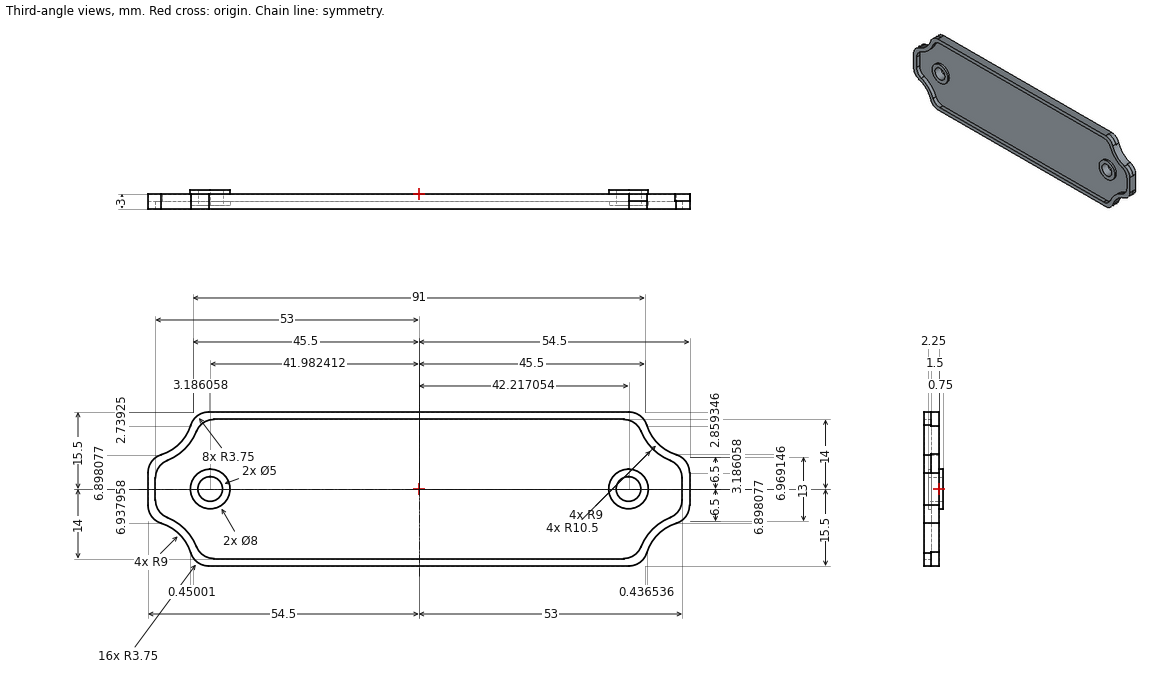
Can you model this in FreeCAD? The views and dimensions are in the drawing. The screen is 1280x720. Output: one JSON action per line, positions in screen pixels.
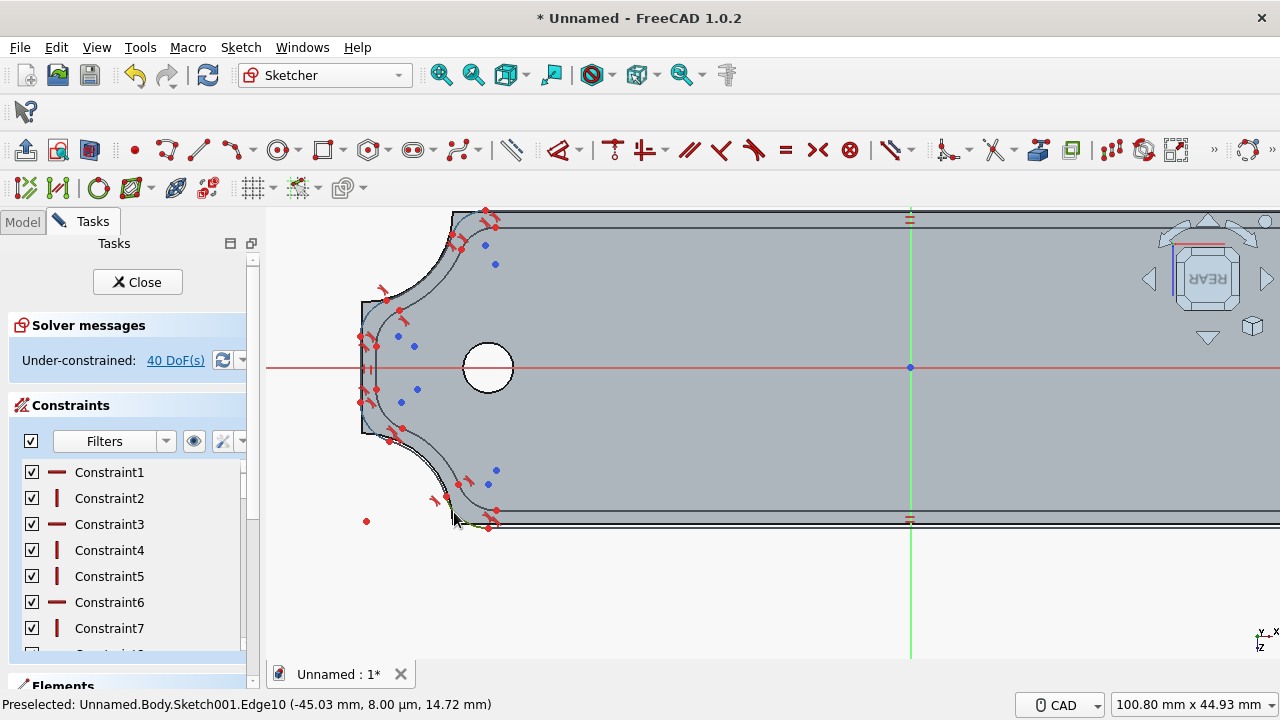
{"action": "scroll", "coordinate": [454, 512], "scroll_direction": "down", "scroll_amount": 3}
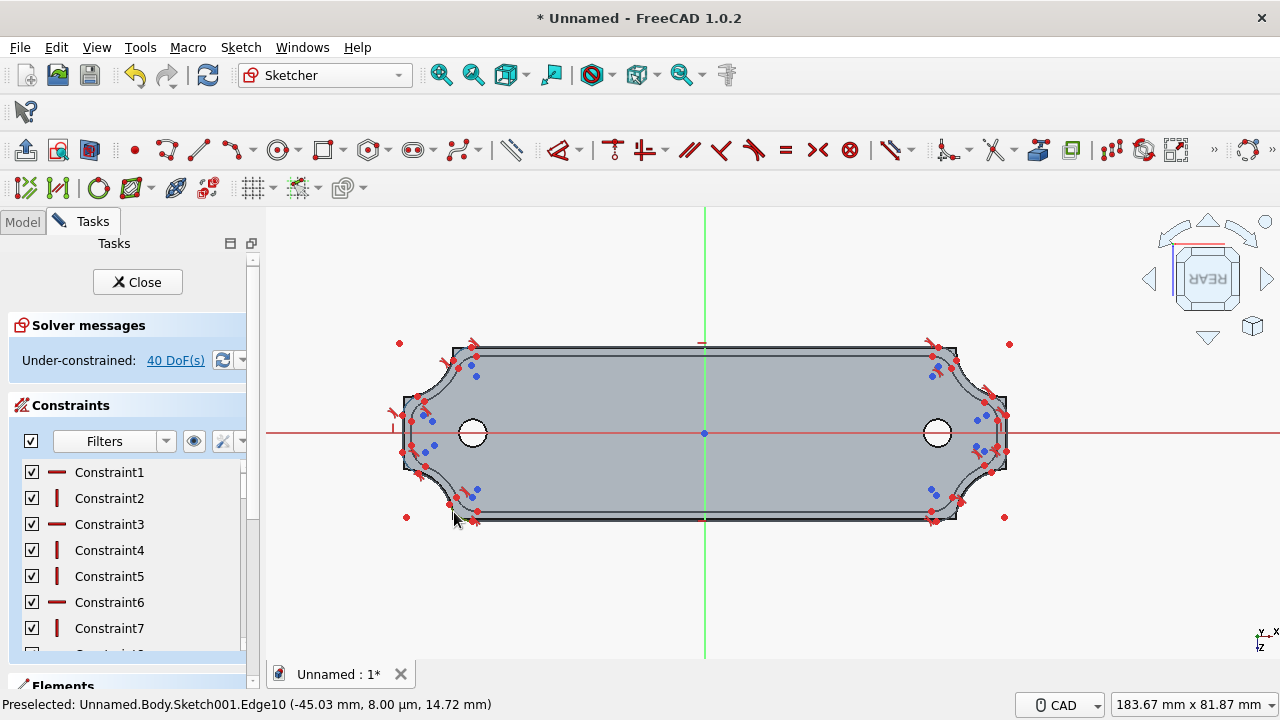
{"action": "scroll", "coordinate": [945, 519], "scroll_direction": "up", "scroll_amount": 2}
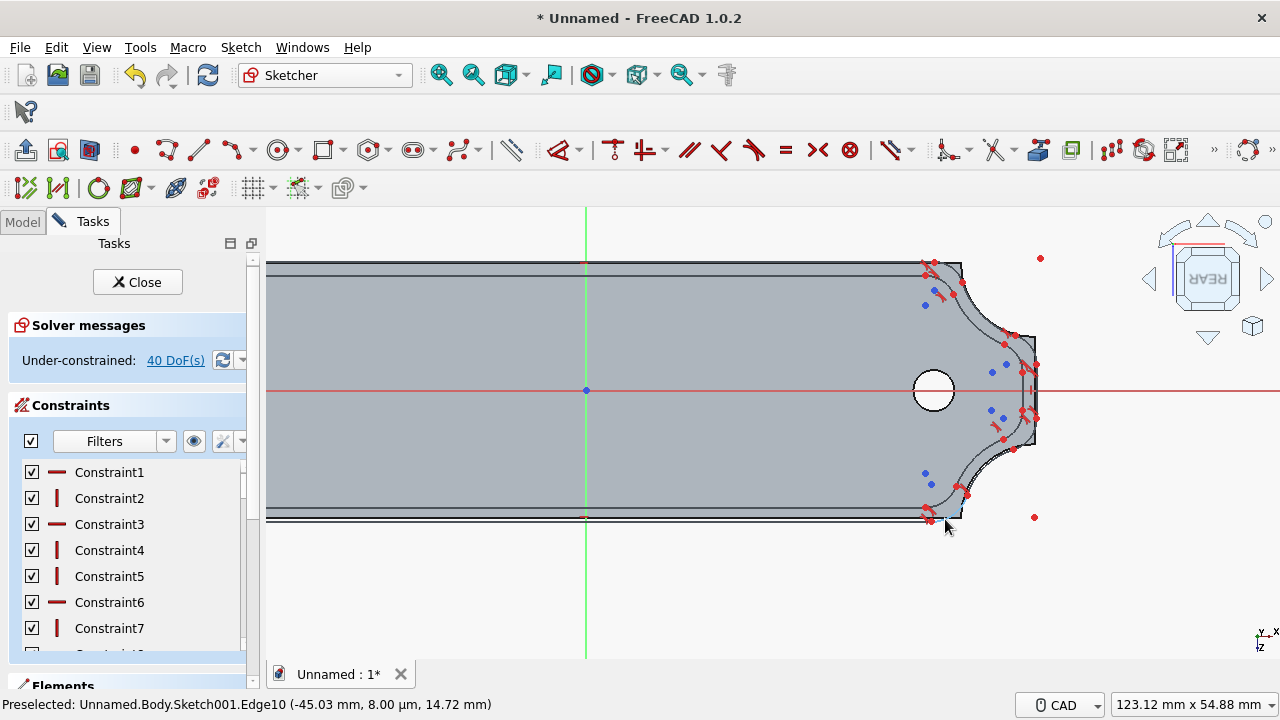
{"action": "left_click", "coordinate": [945, 519]}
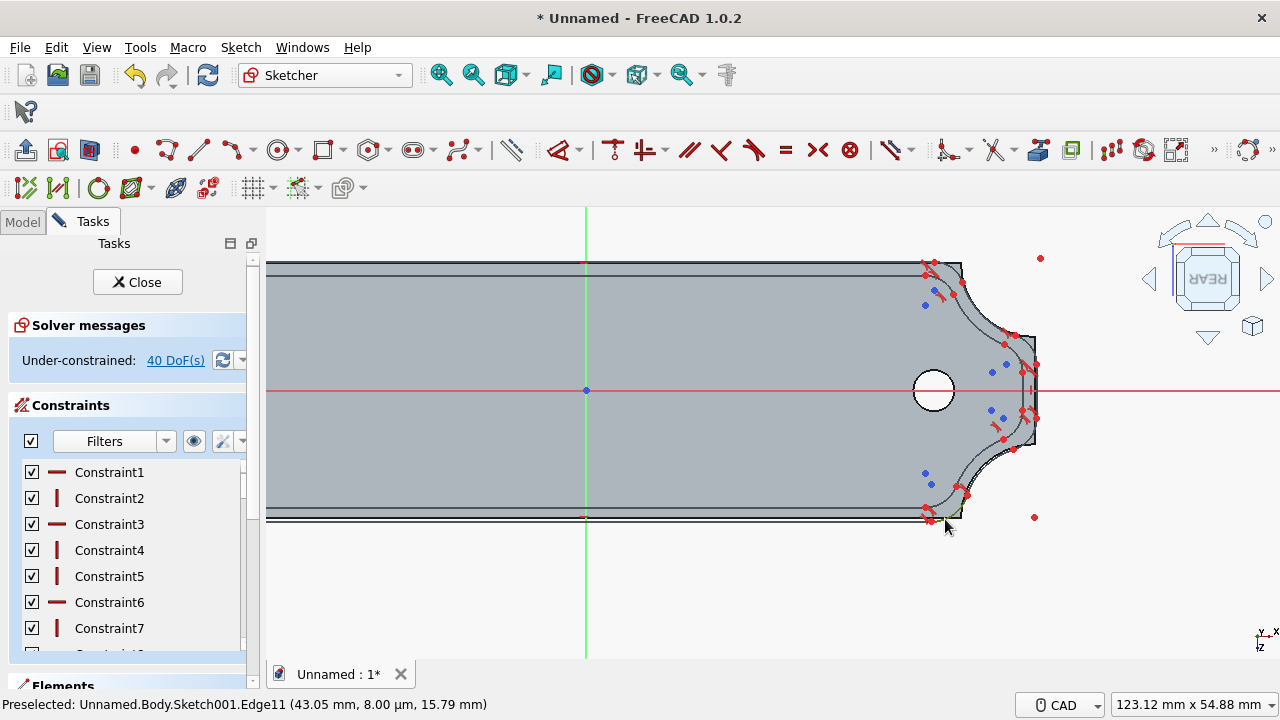
{"action": "left_click", "coordinate": [1025, 444]}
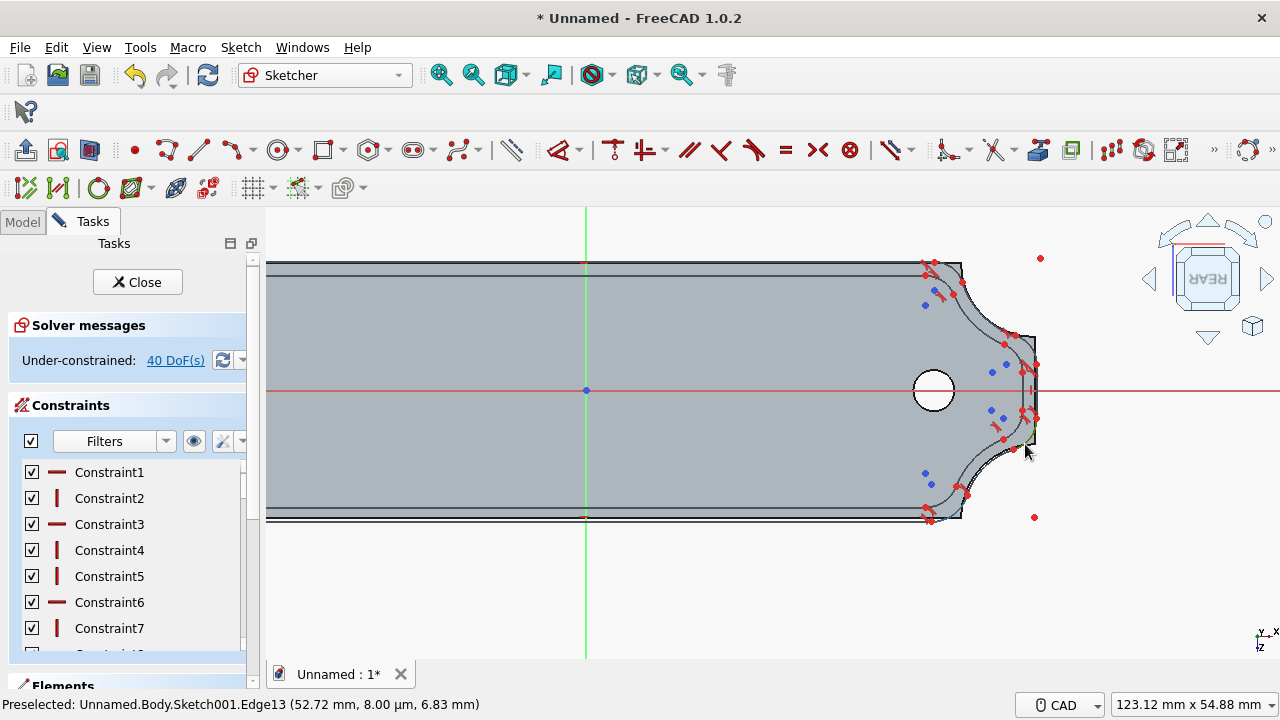
{"action": "left_click", "coordinate": [1035, 354]}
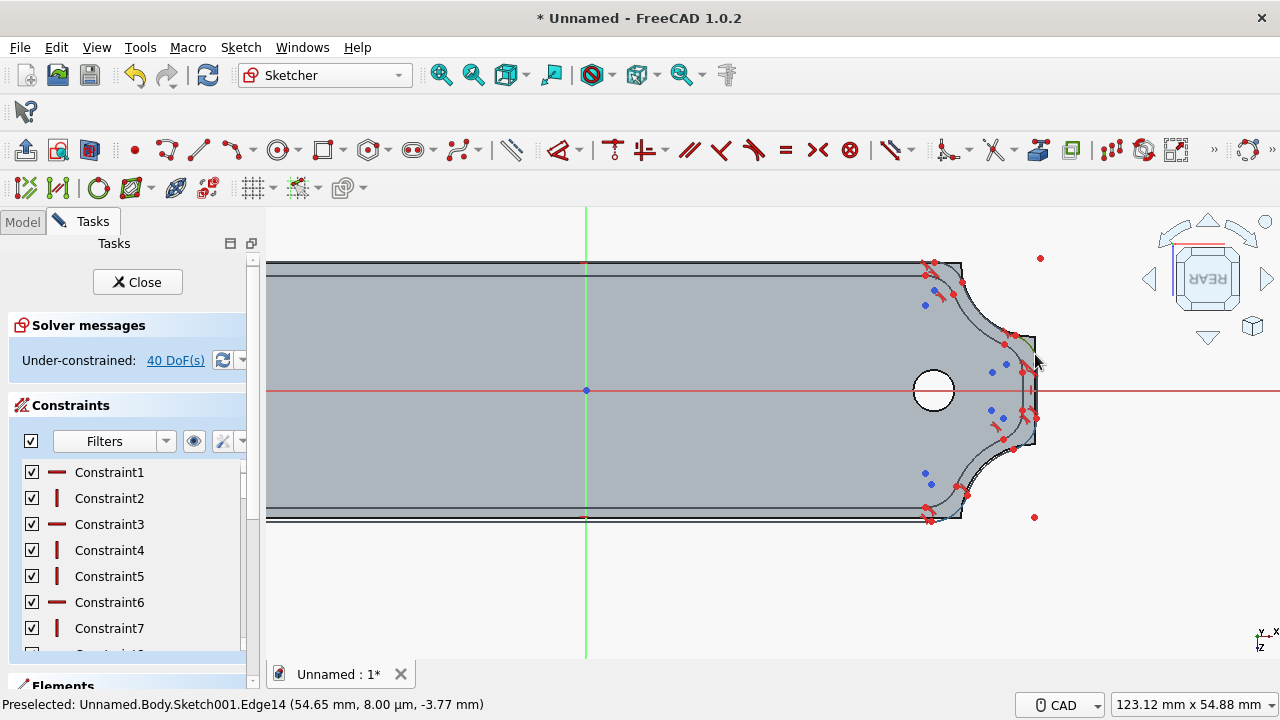
{"action": "scroll", "coordinate": [957, 273], "scroll_direction": "up", "scroll_amount": 2}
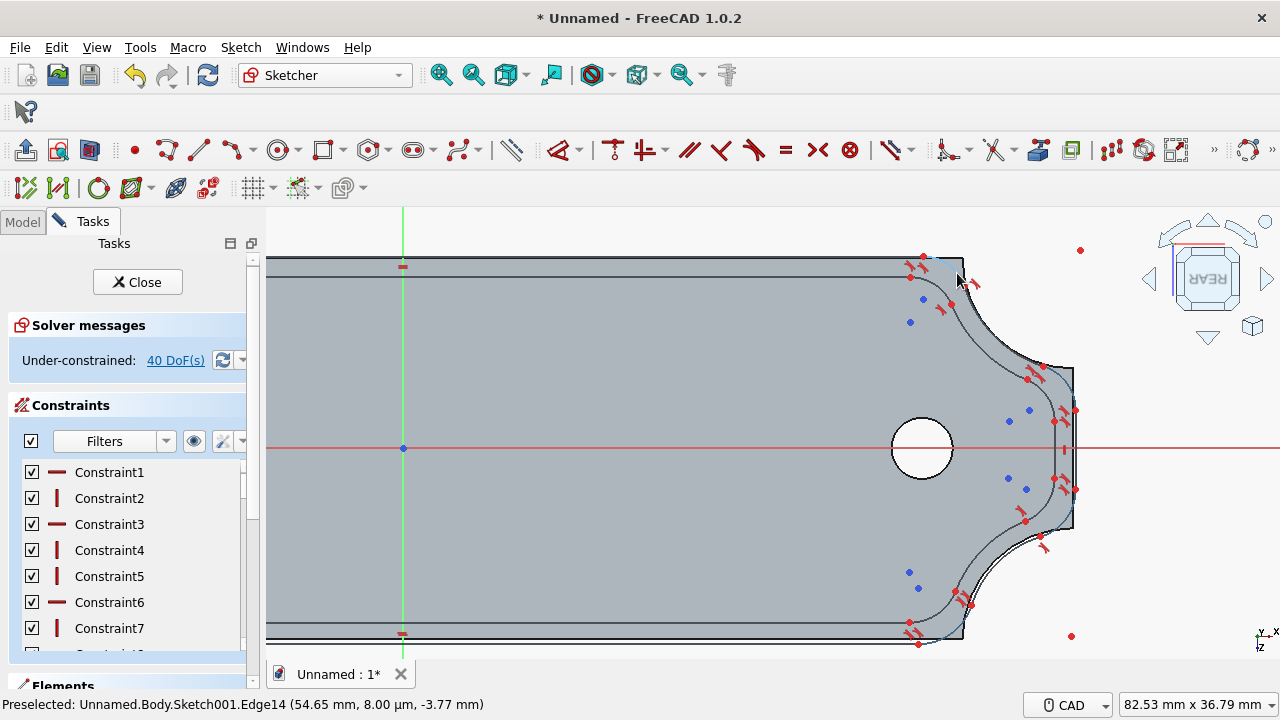
{"action": "left_click", "coordinate": [957, 273]}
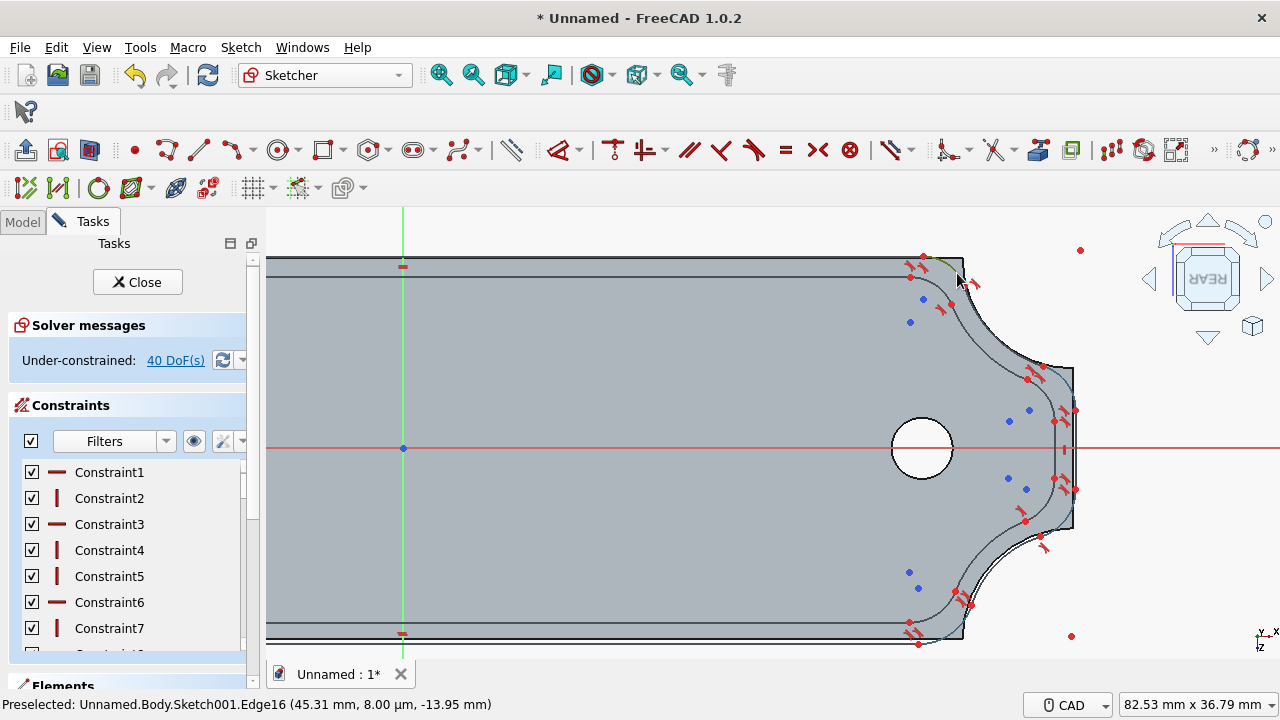
{"action": "left_click", "coordinate": [1039, 512]}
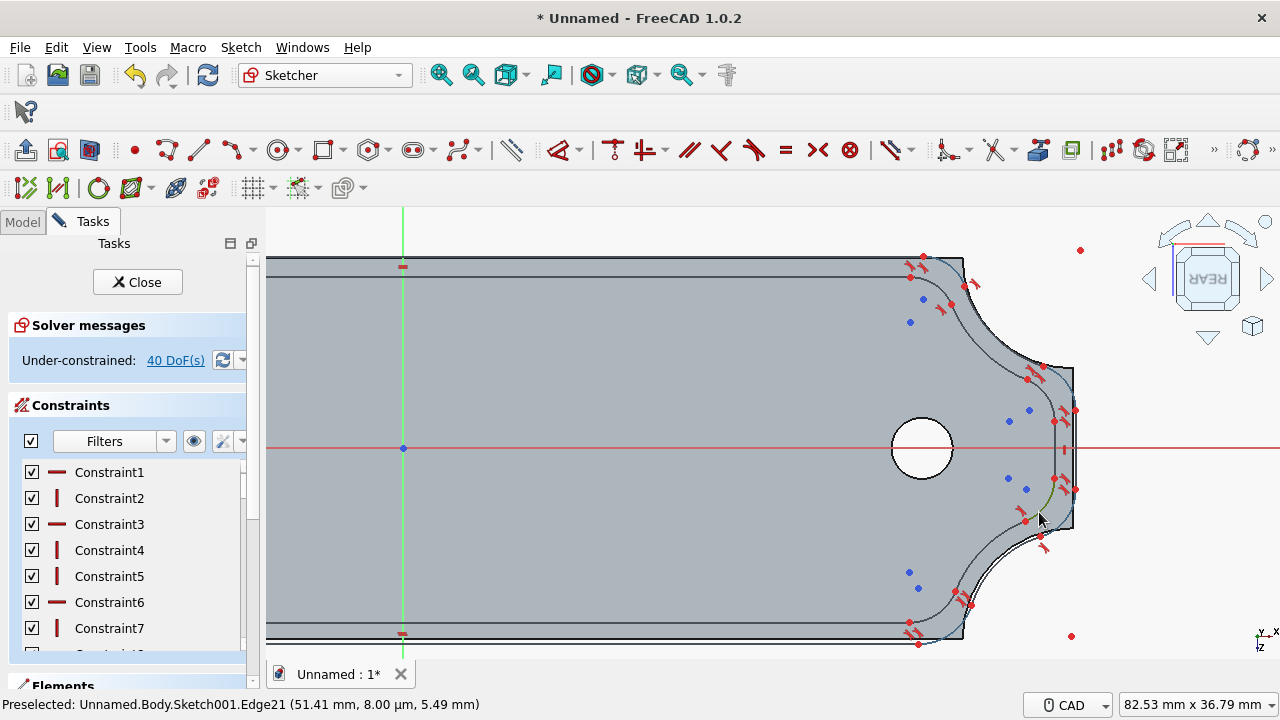
{"action": "left_click", "coordinate": [927, 620]}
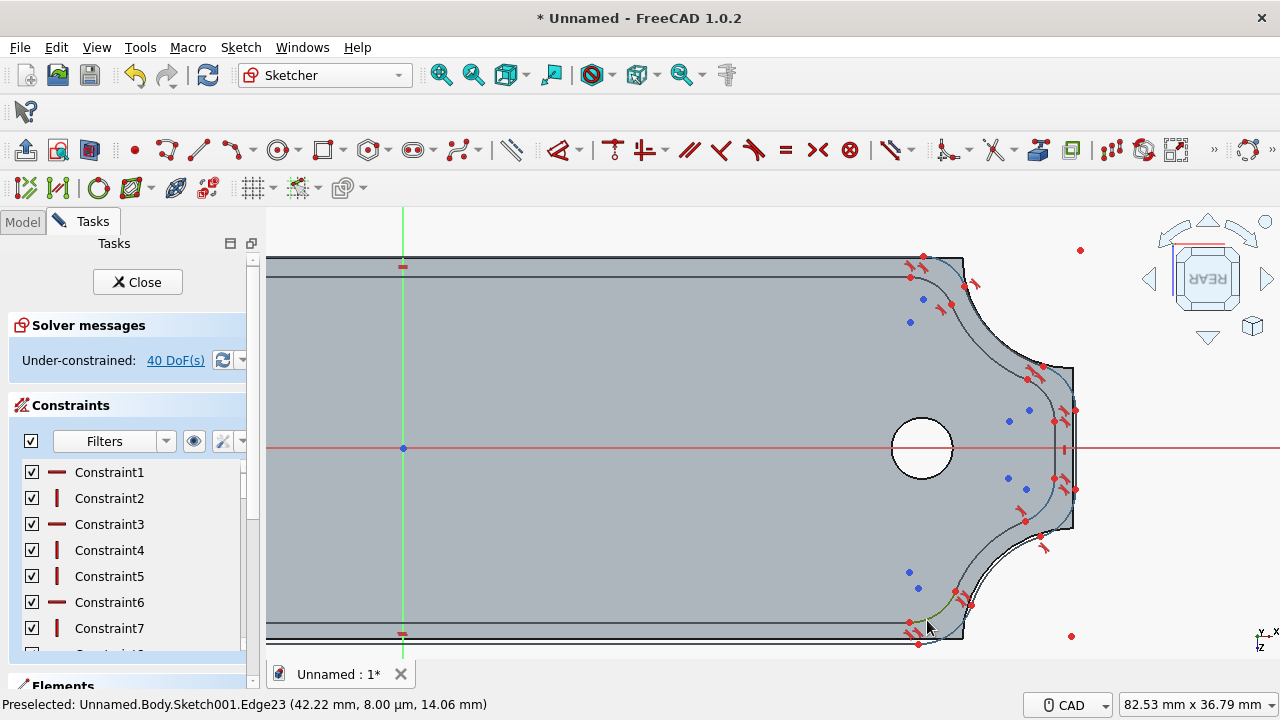
{"action": "scroll", "coordinate": [950, 420], "scroll_direction": "down", "scroll_amount": 4}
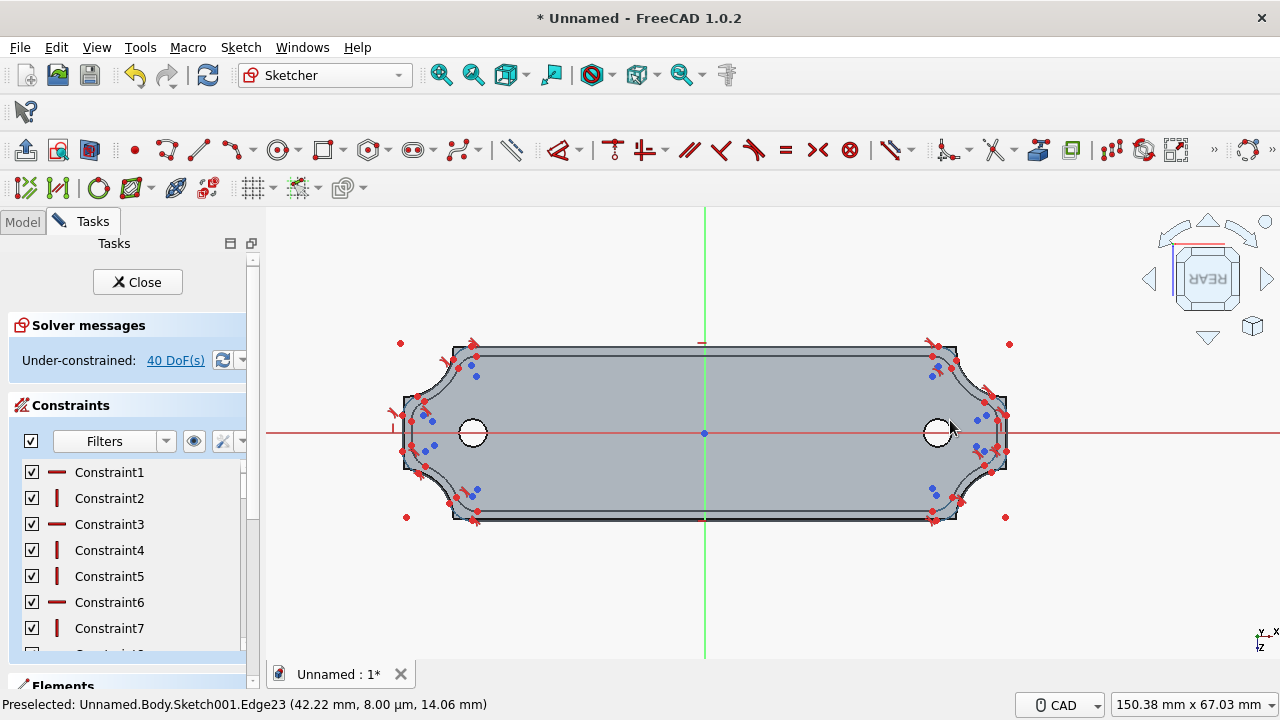
{"action": "scroll", "coordinate": [461, 504], "scroll_direction": "up", "scroll_amount": 3}